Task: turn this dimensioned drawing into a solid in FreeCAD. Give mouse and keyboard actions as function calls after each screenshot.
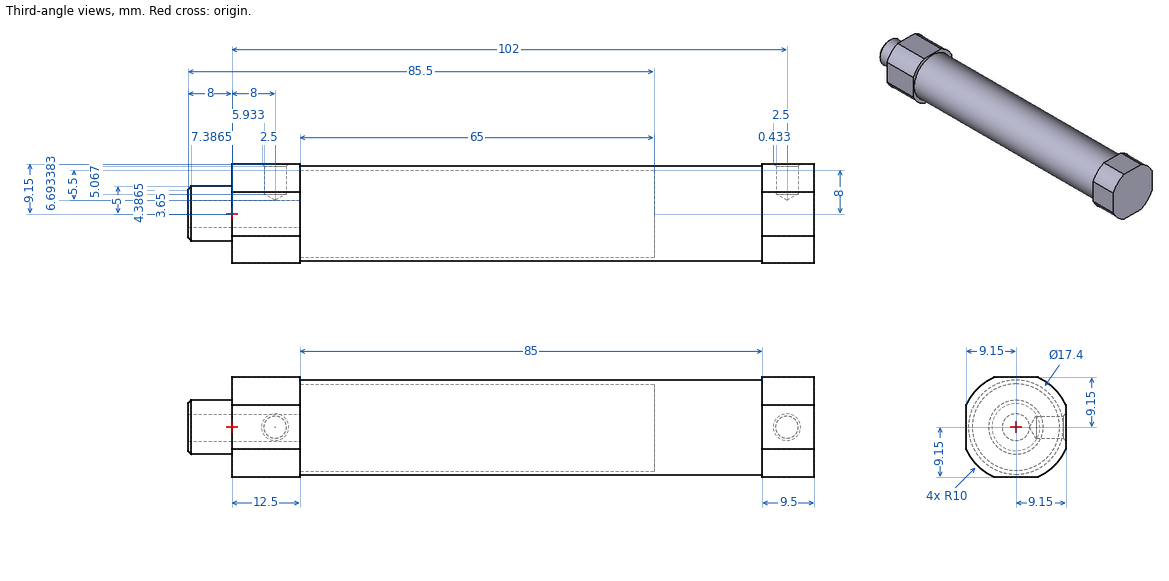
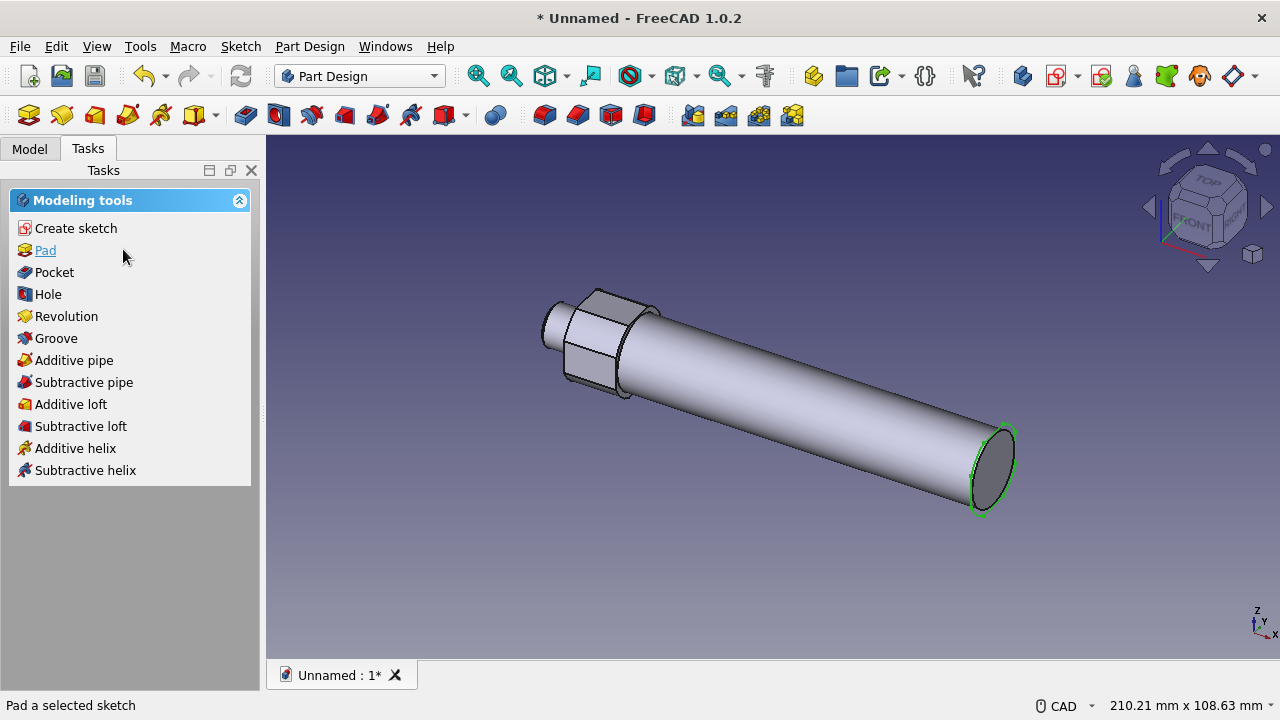
click(29, 116)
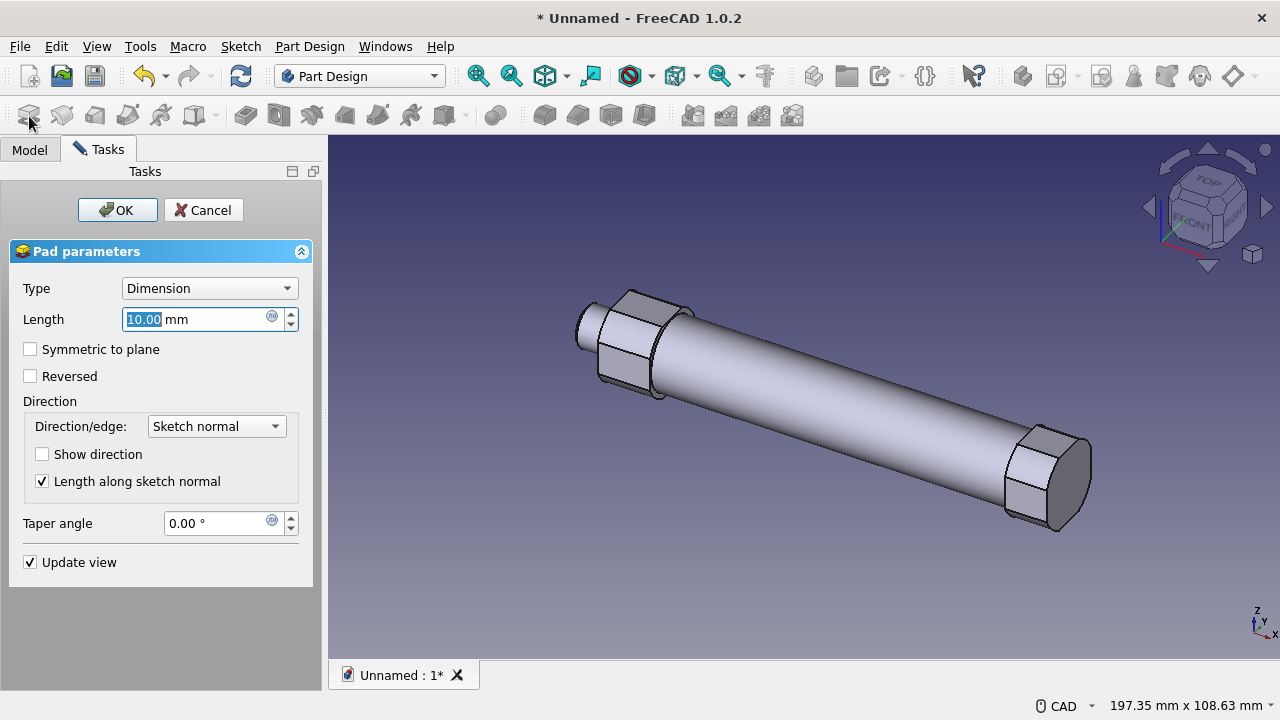
text(9.5)
key(Tab)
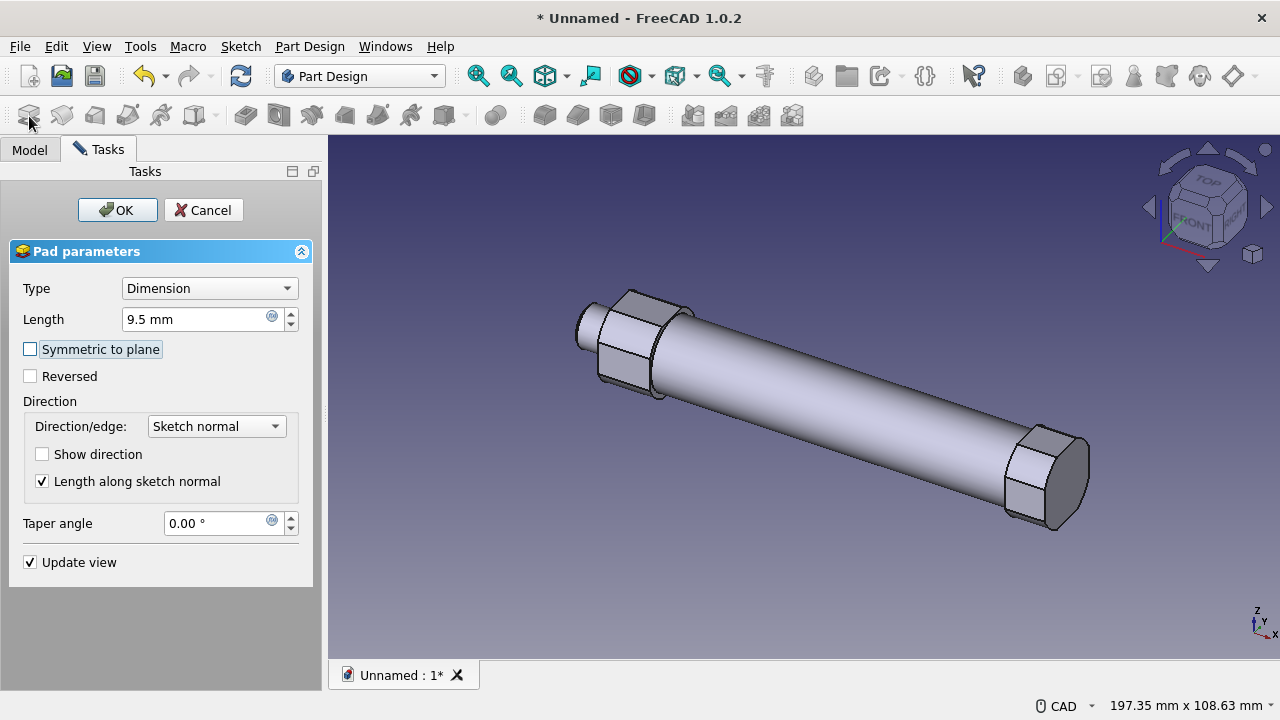
click(118, 210)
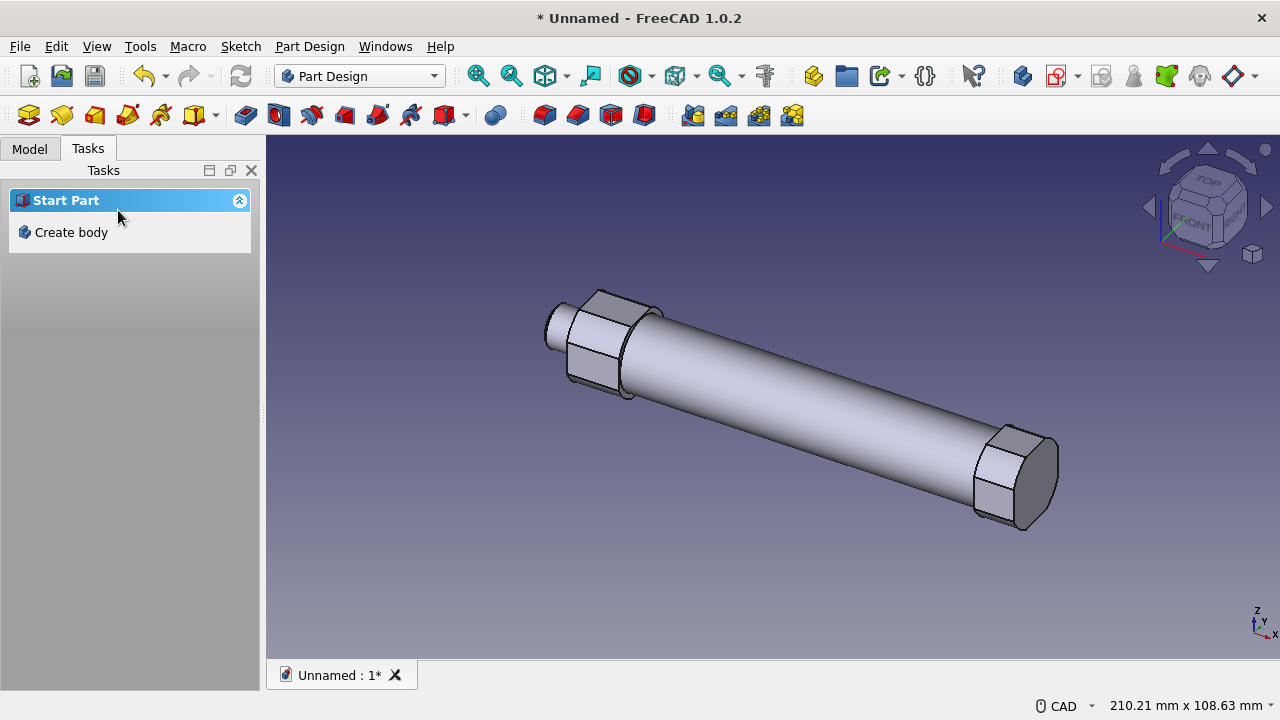
click(1056, 76)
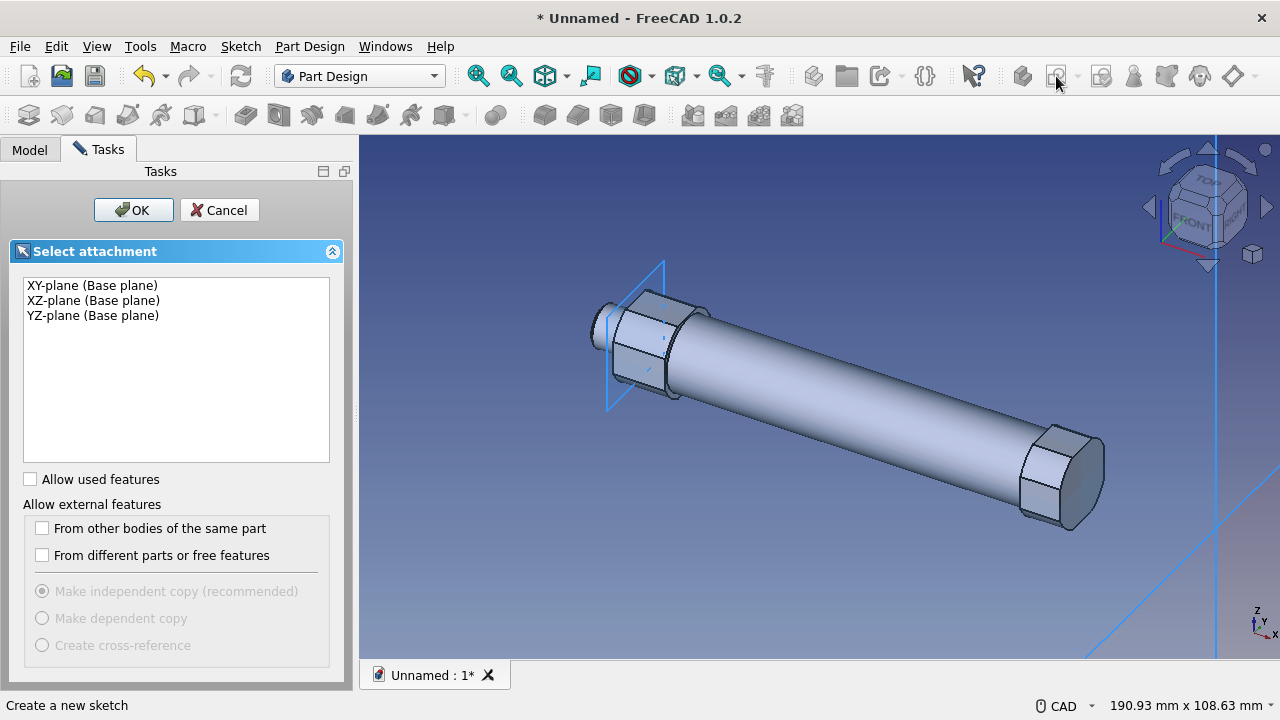
click(84, 286)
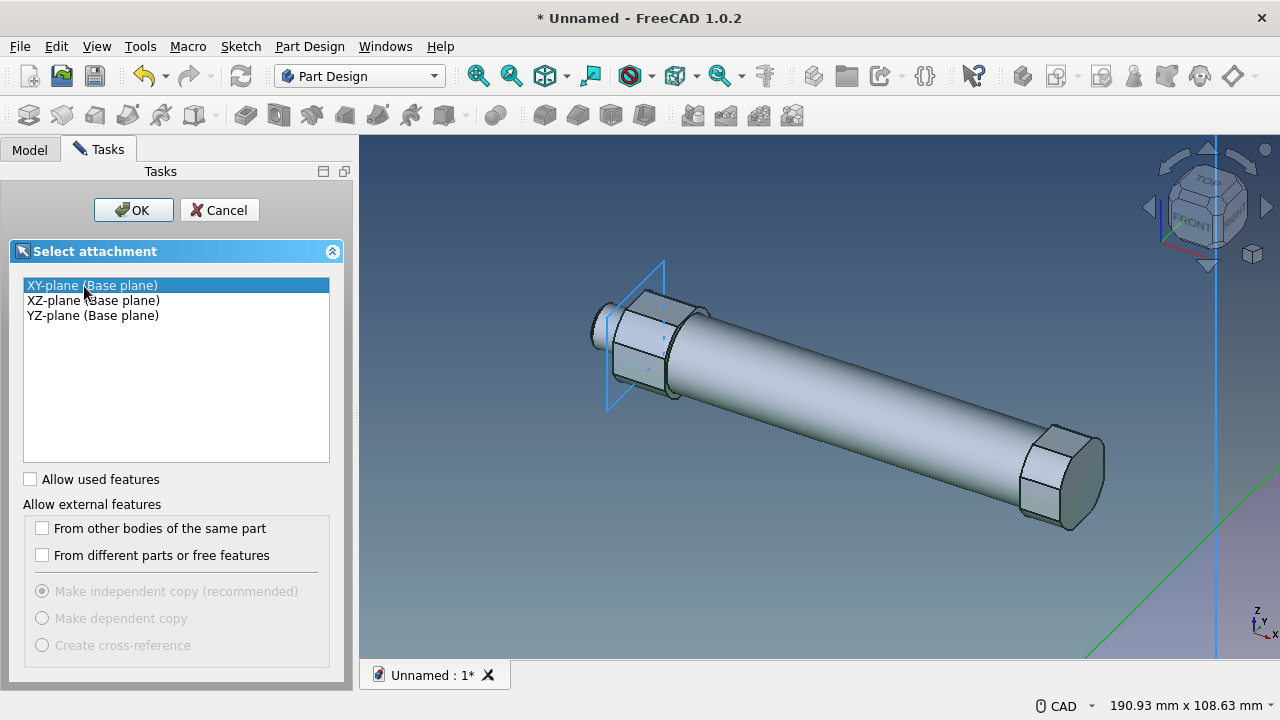
click(134, 210)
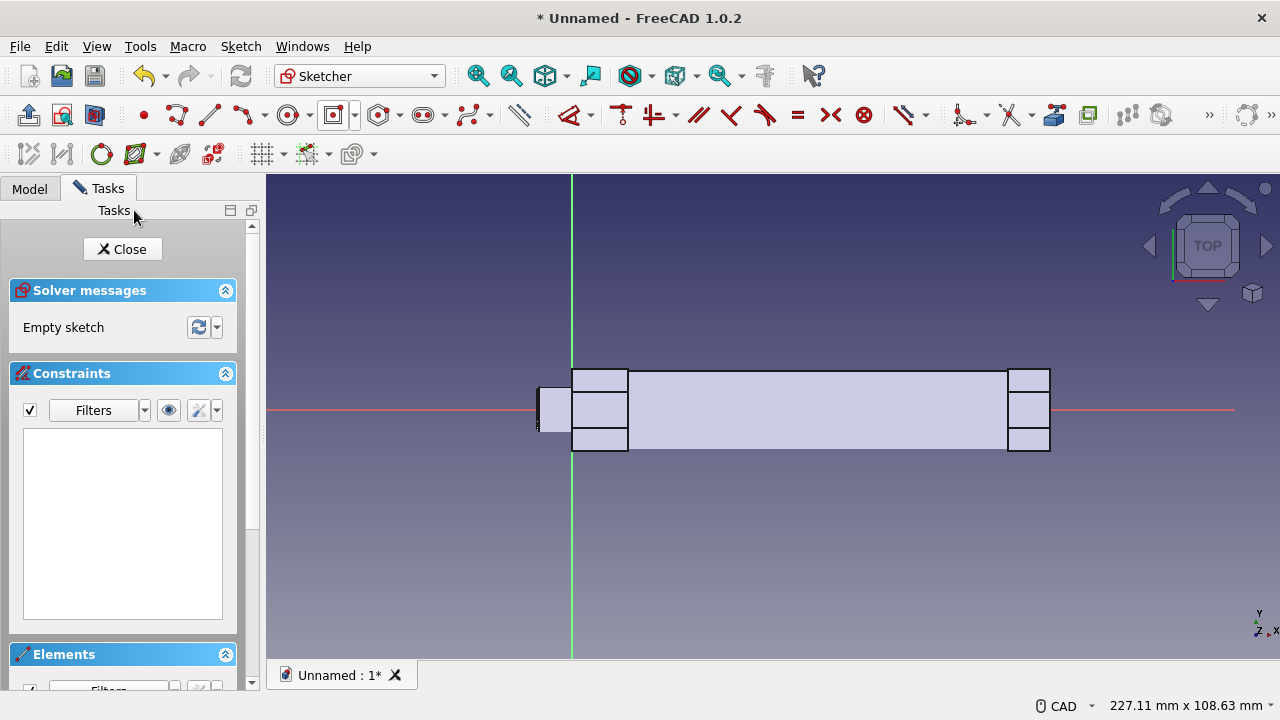
click(95, 116)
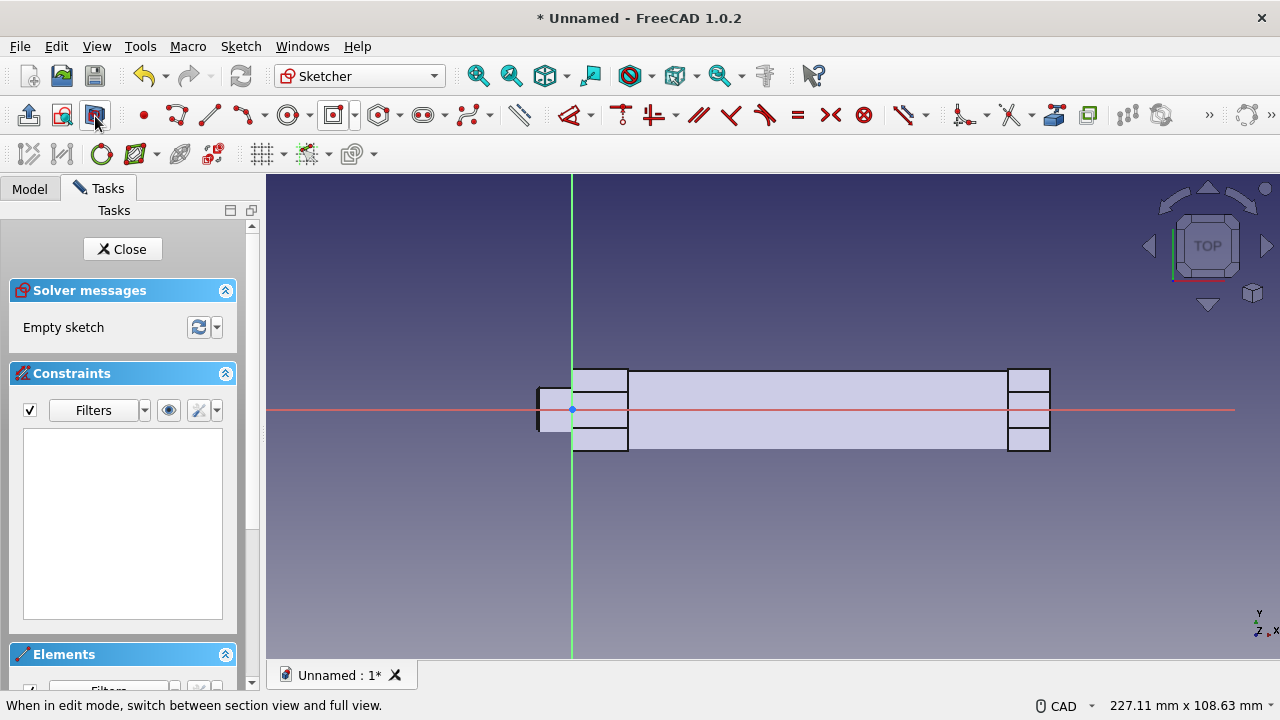
scroll(572, 386, up, 10)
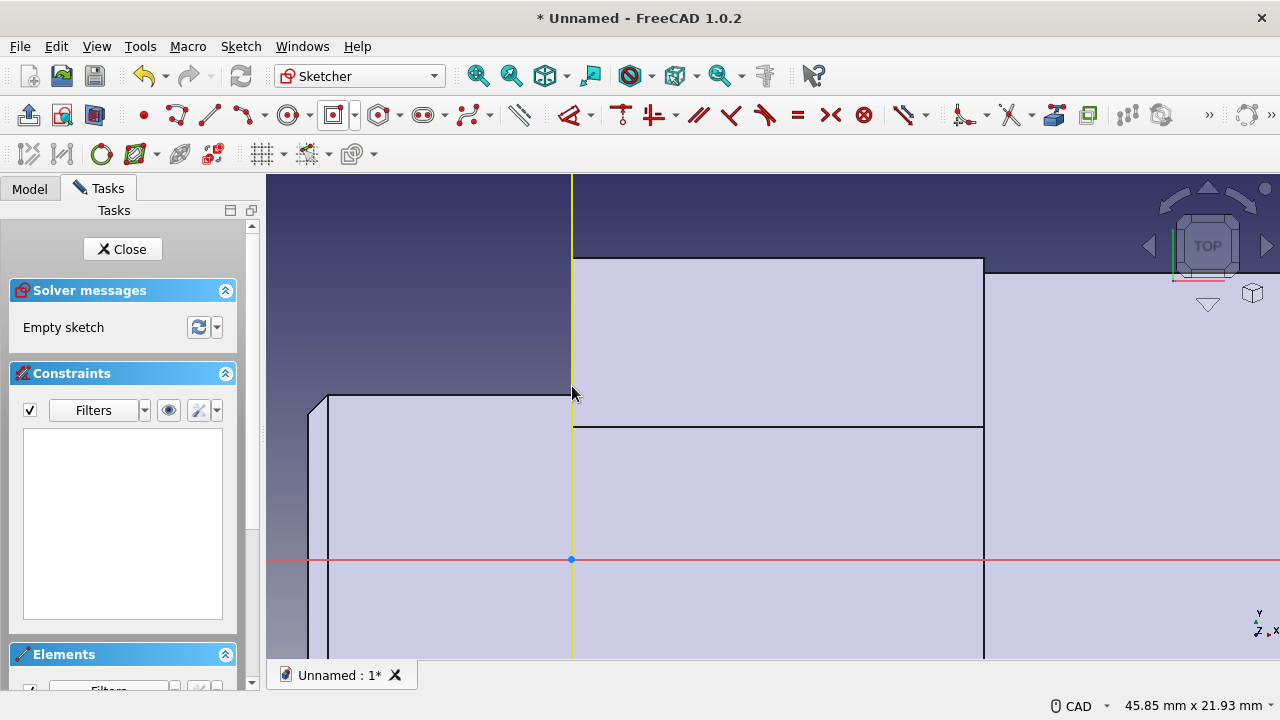
click(177, 116)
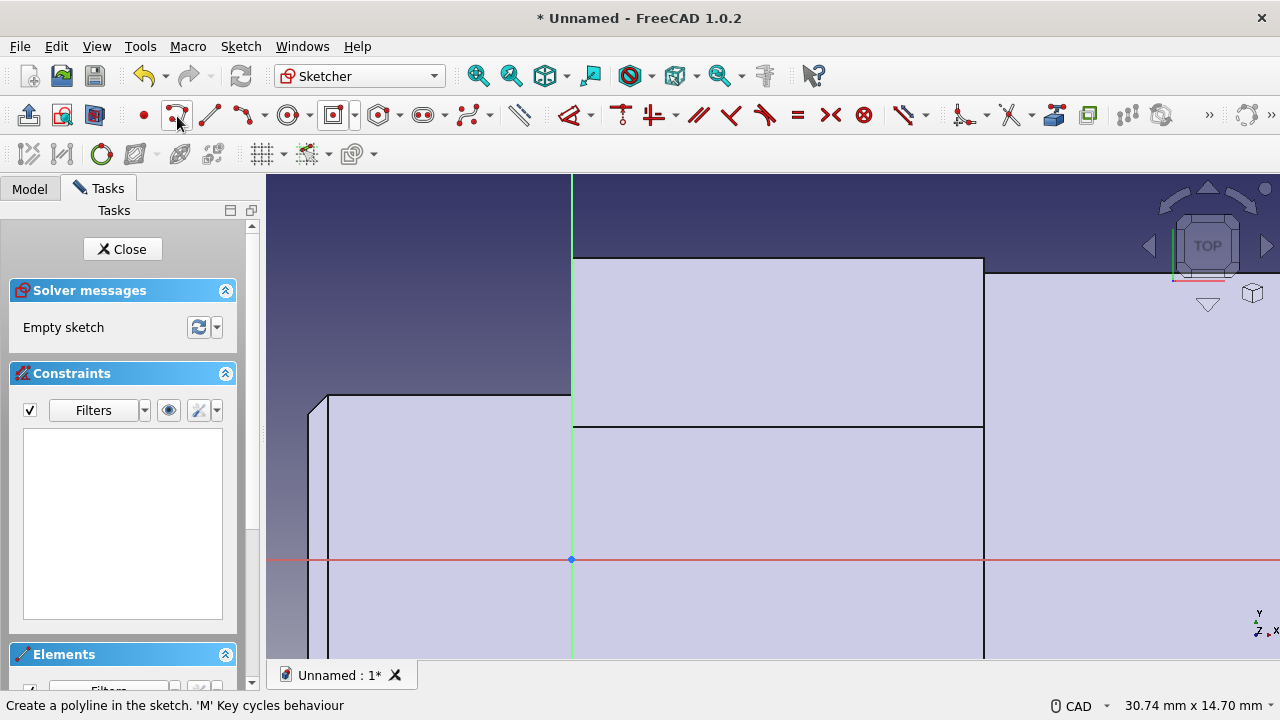
click(768, 439)
click(836, 479)
click(836, 258)
click(753, 258)
click(768, 272)
click(768, 440)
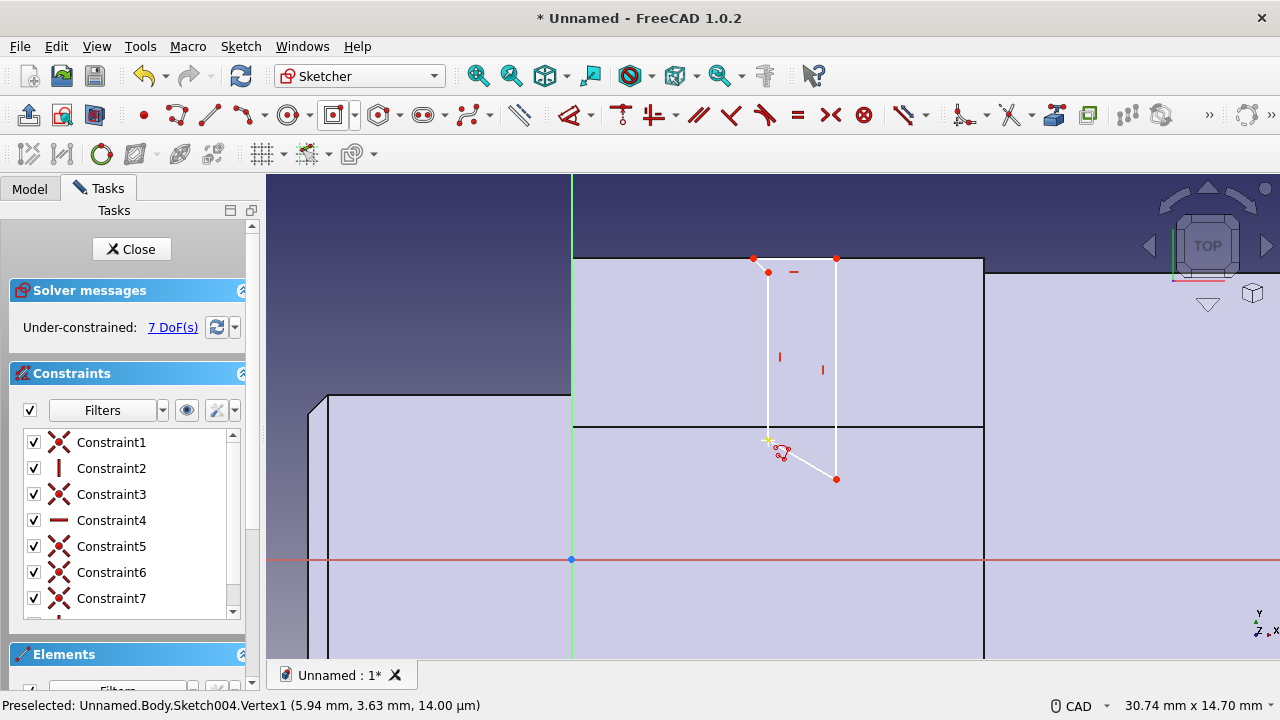
click(210, 116)